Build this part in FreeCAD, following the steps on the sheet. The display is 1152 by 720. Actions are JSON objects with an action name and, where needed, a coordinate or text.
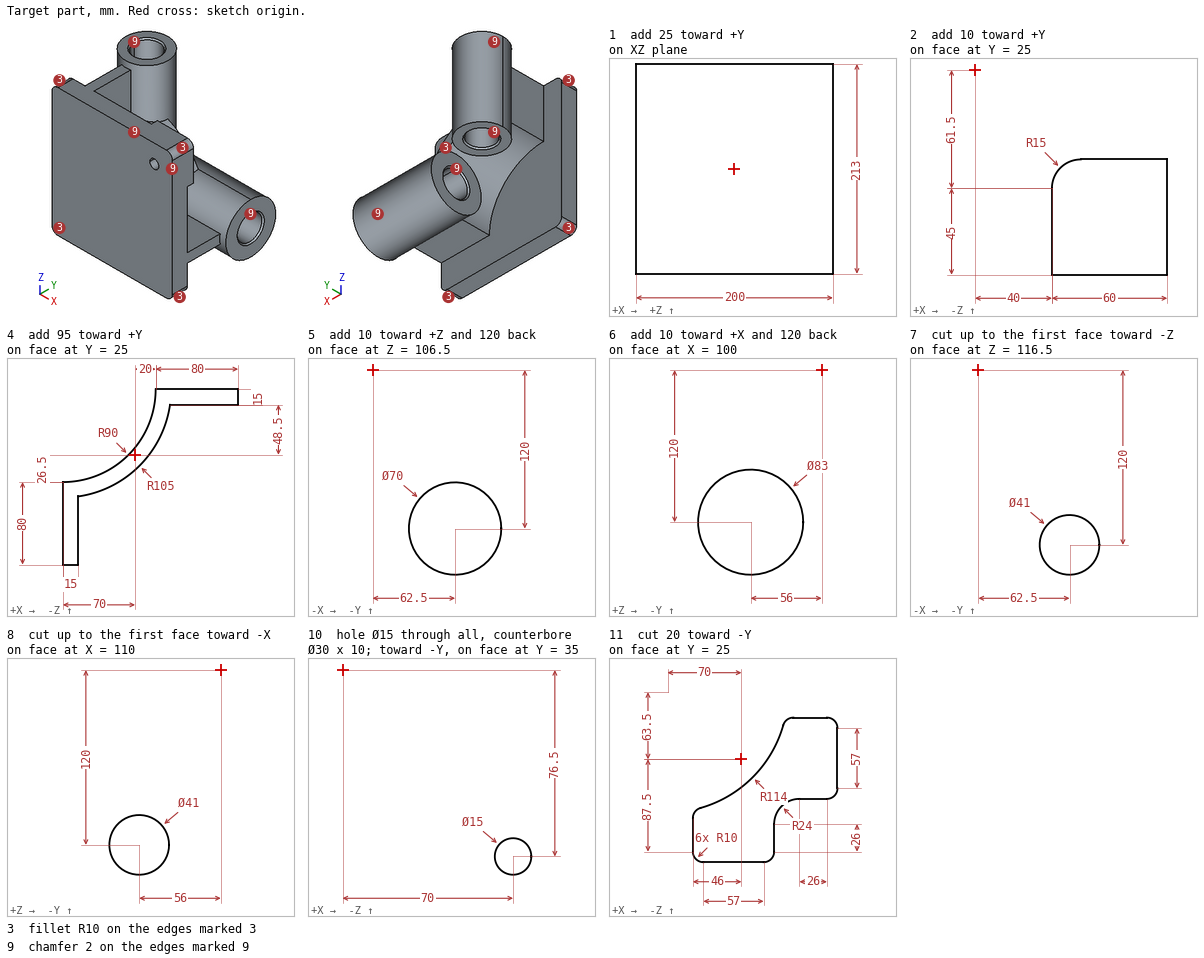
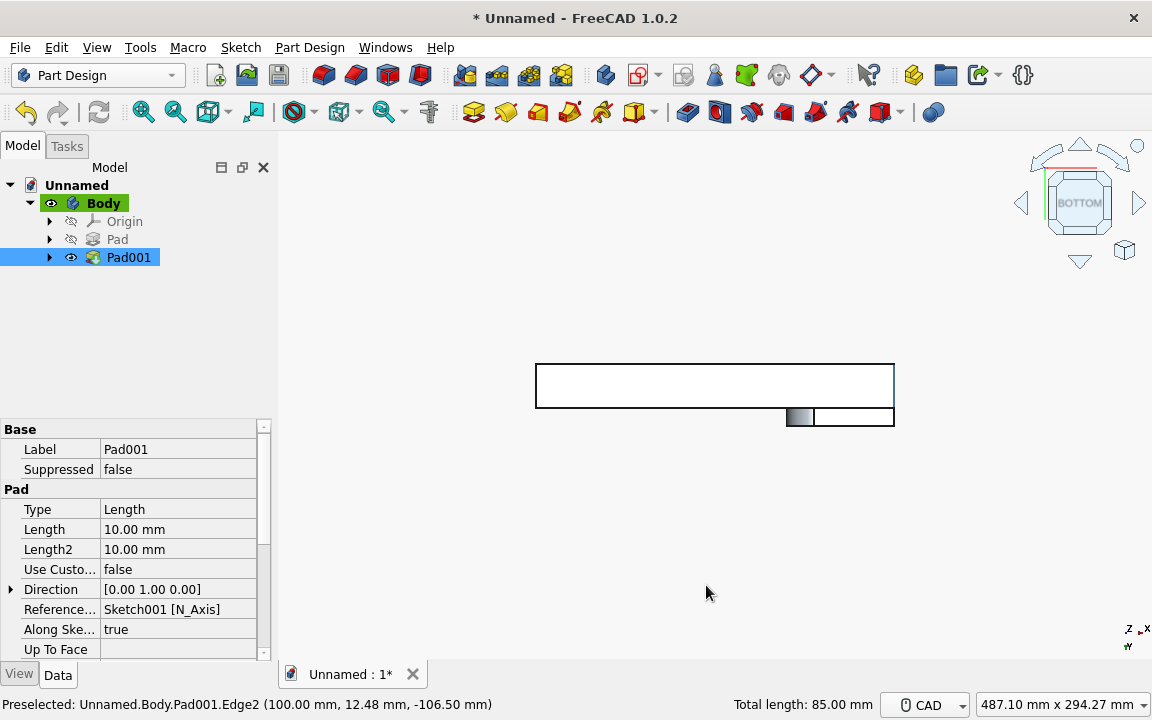
{"action": "left_click", "coordinate": [144, 112]}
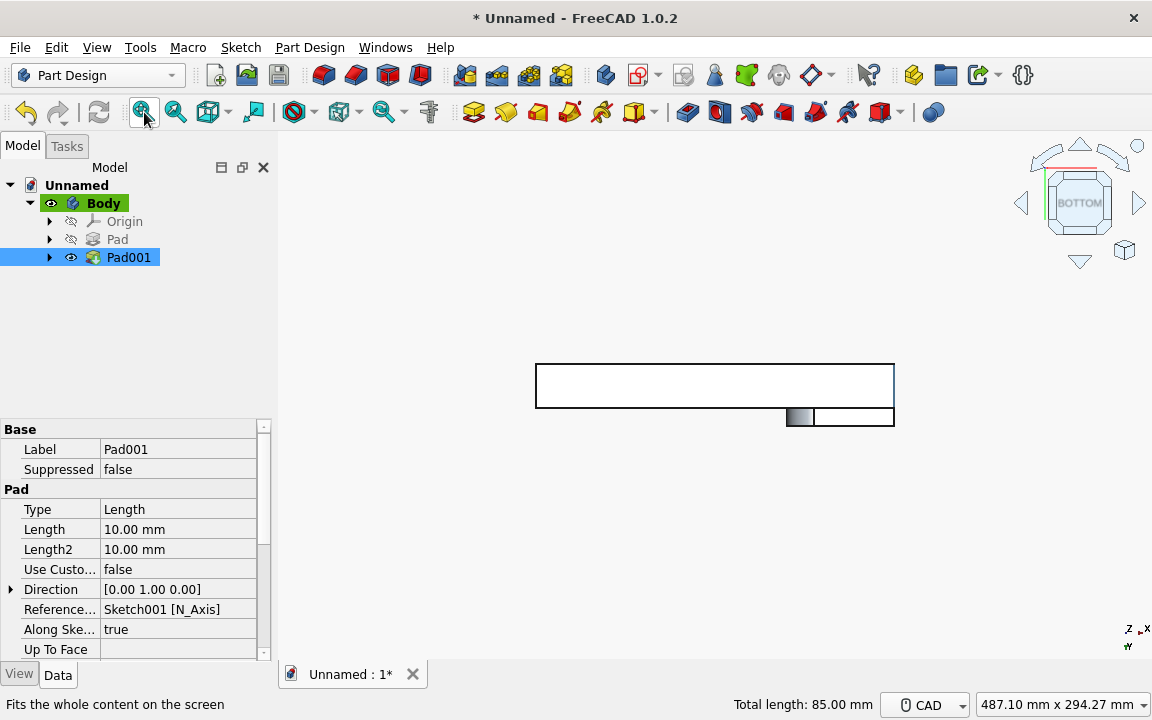
{"action": "left_click", "coordinate": [536, 385], "text": "ctrl"}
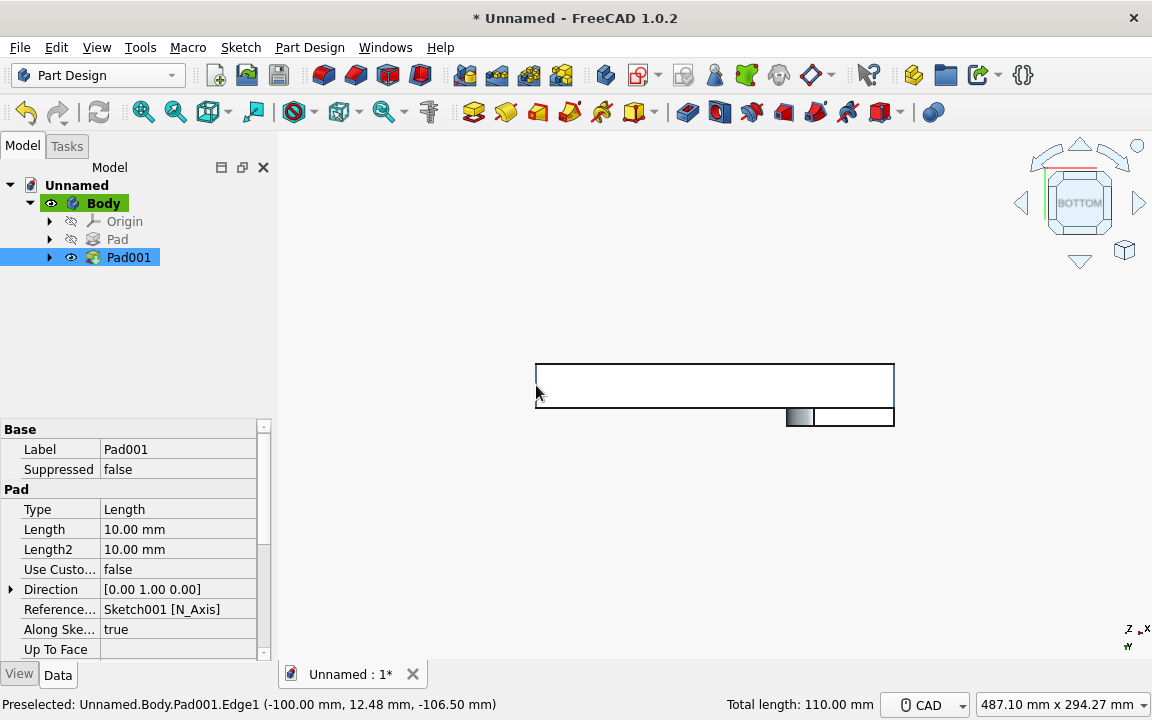
{"action": "left_click", "coordinate": [324, 76]}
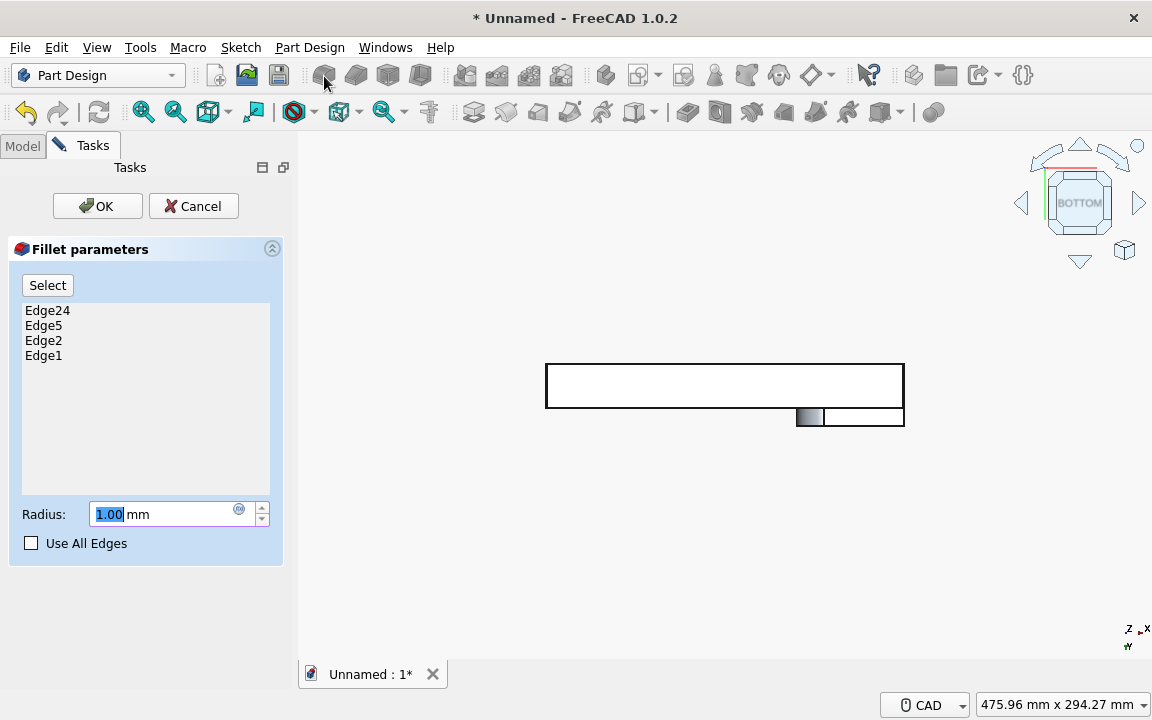
{"action": "type", "text": "10"}
{"action": "key", "text": "Tab"}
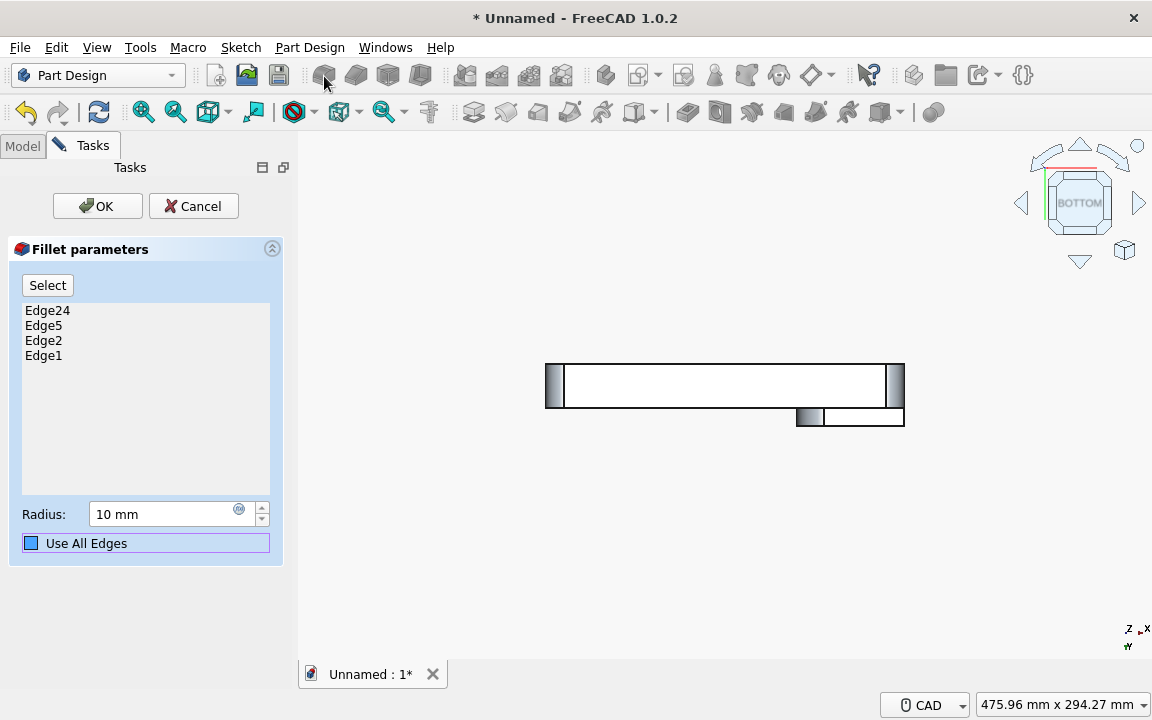
{"action": "left_click", "coordinate": [98, 206]}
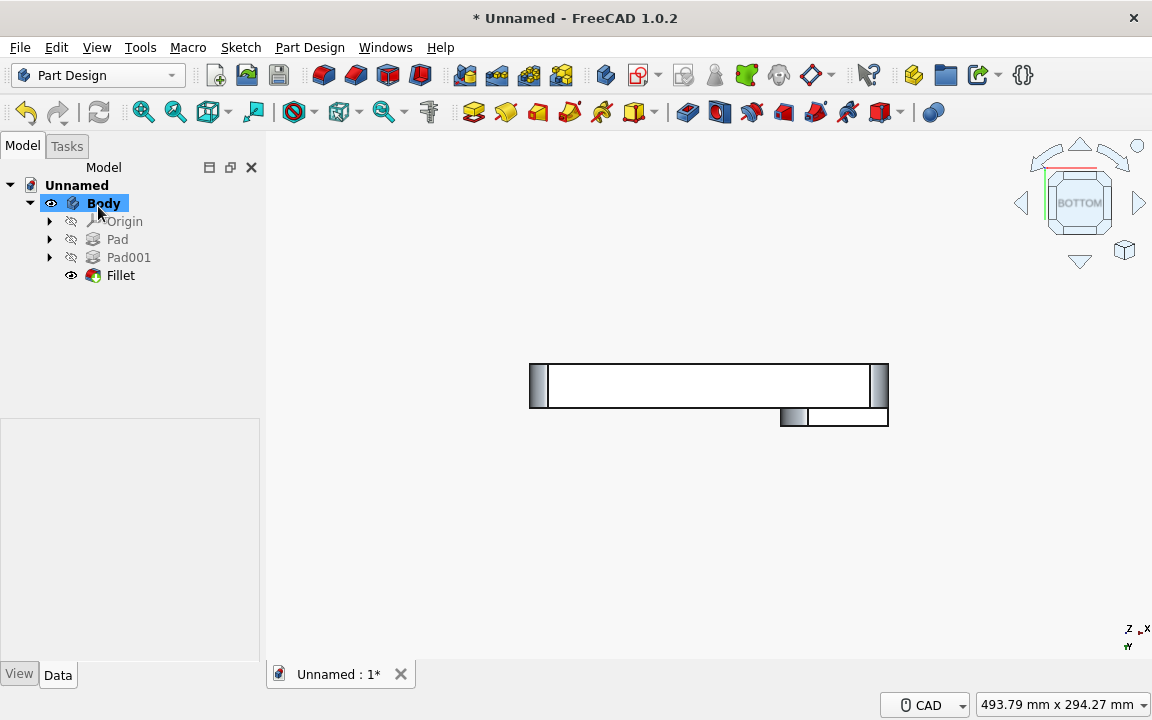
{"action": "left_click", "coordinate": [144, 112]}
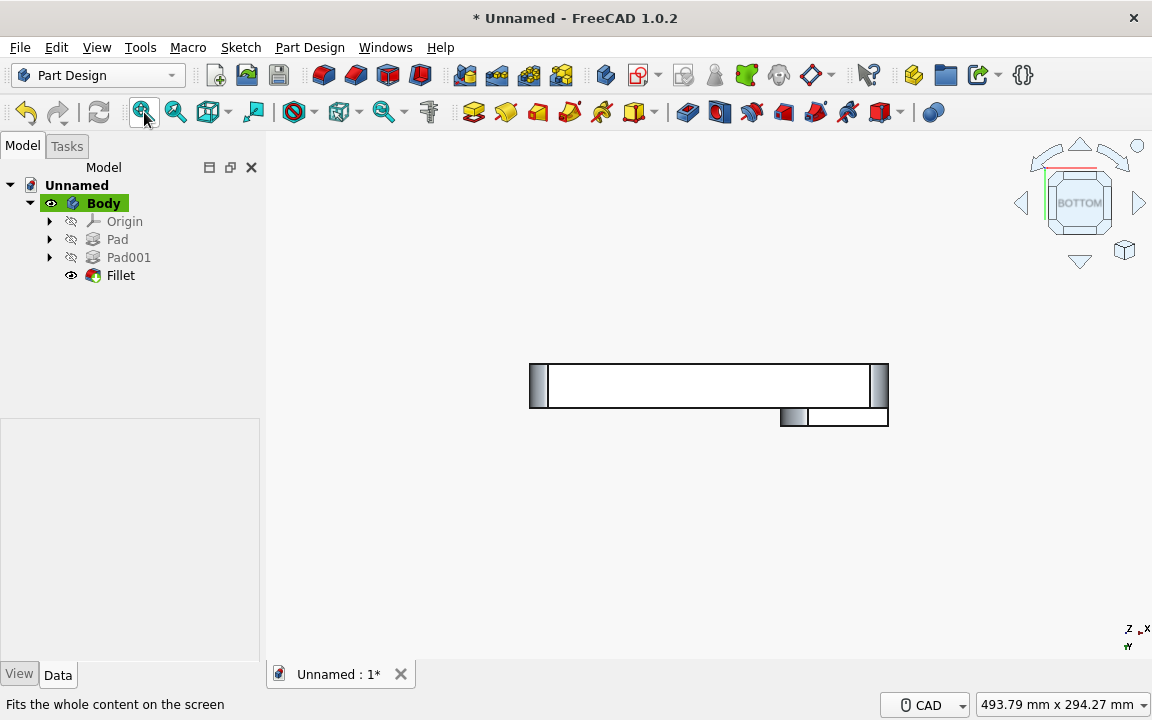
{"action": "key", "text": "4"}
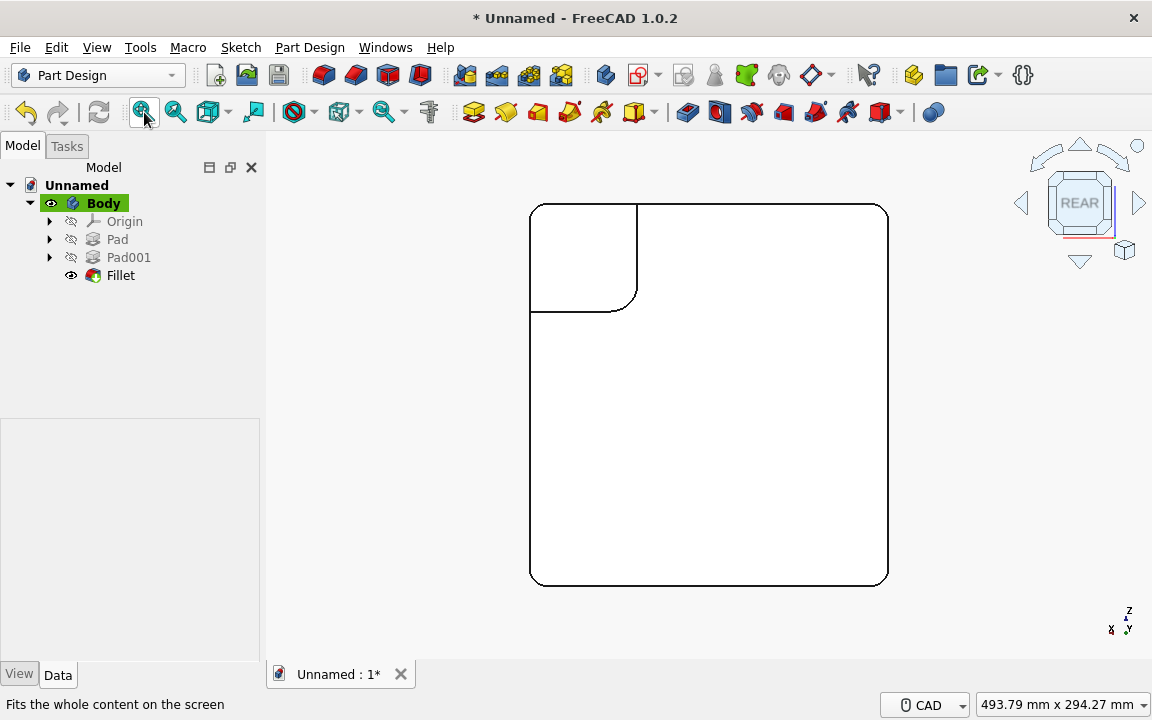
{"action": "left_click", "coordinate": [709, 449]}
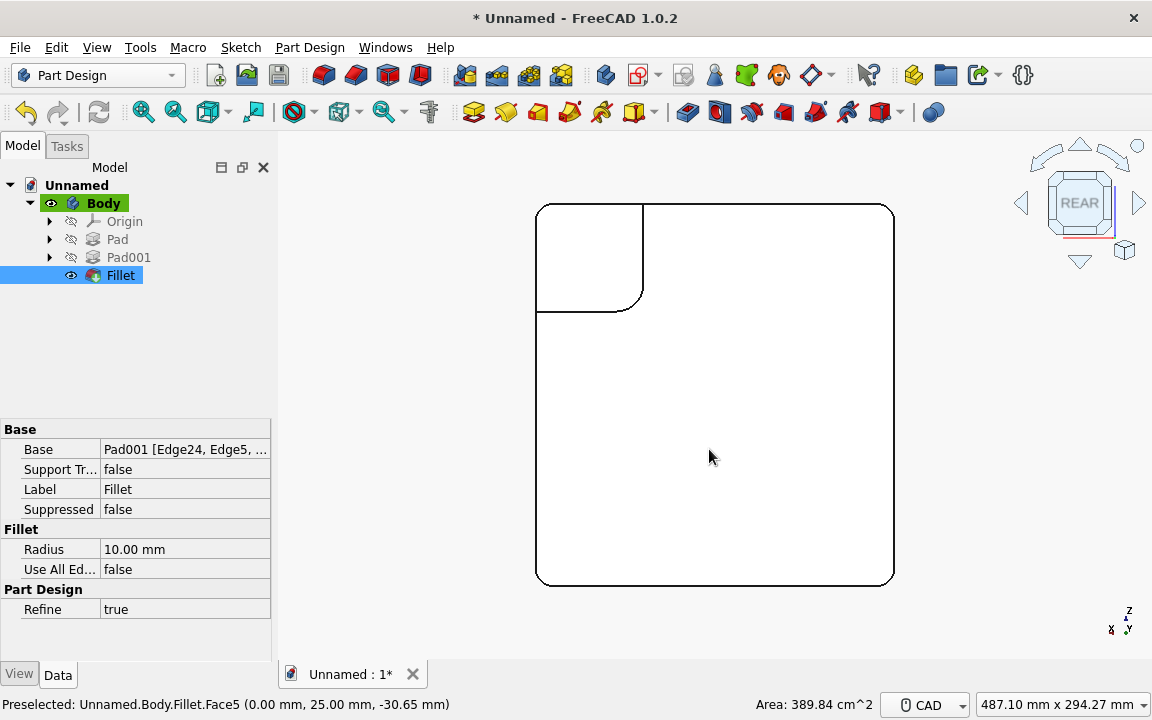
{"action": "left_click", "coordinate": [638, 76]}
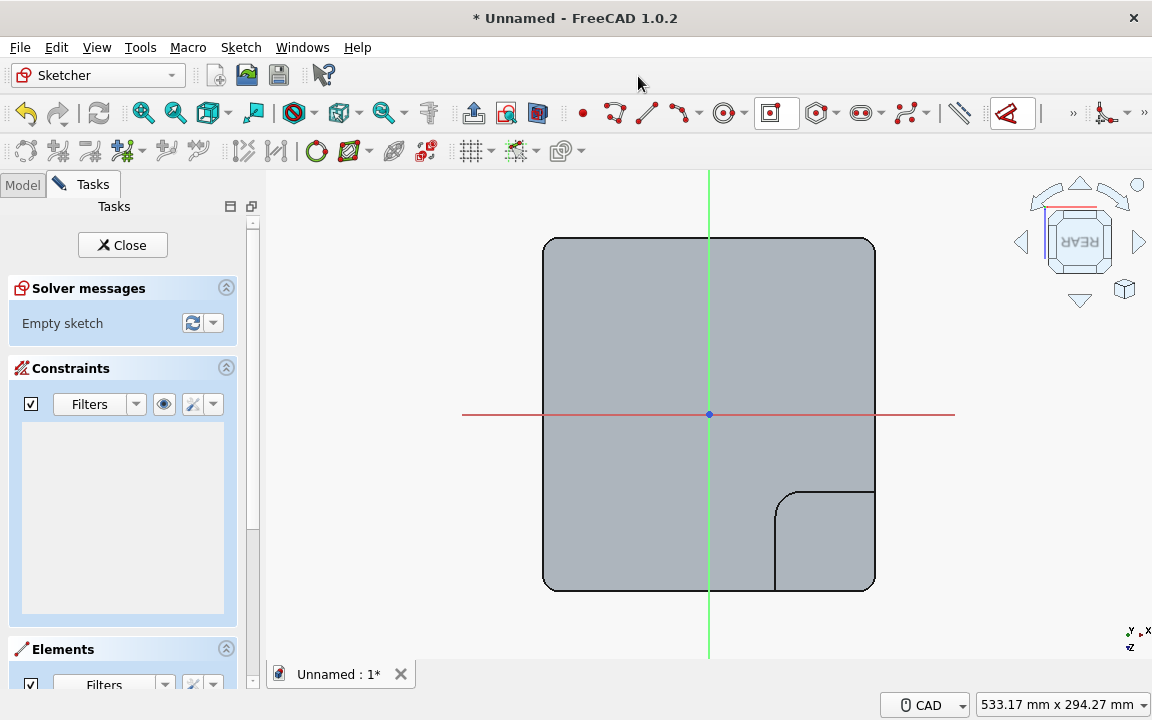
{"action": "left_click", "coordinate": [538, 114]}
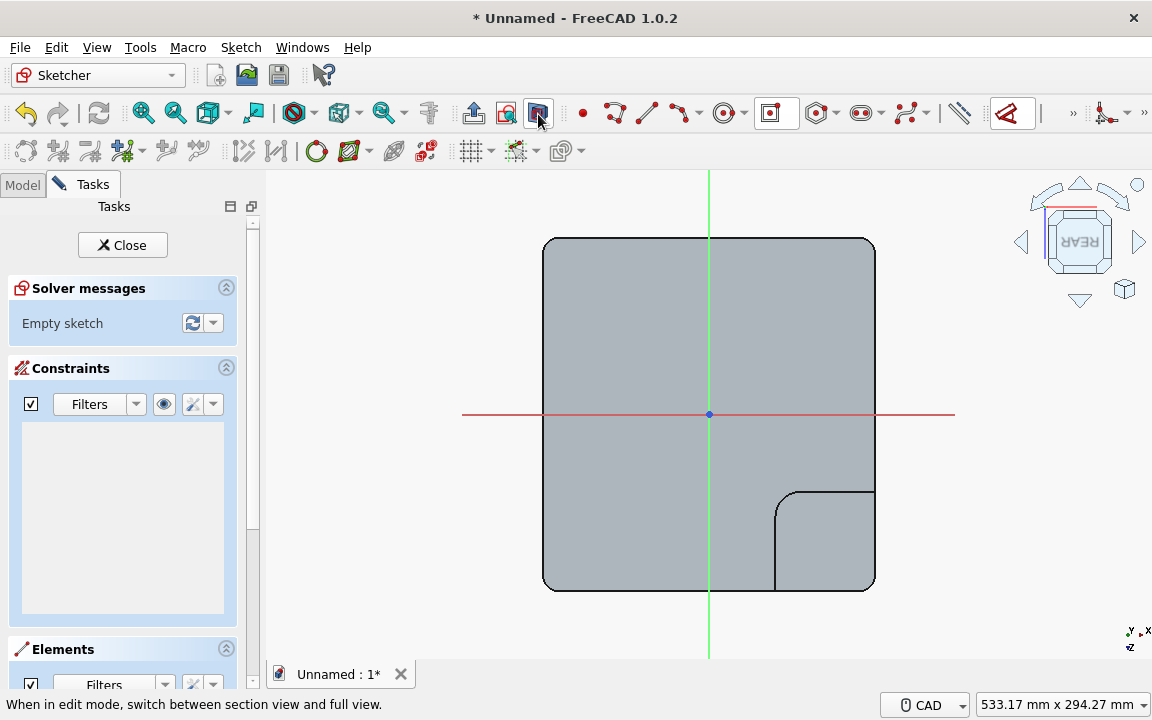
{"action": "left_click", "coordinate": [616, 114]}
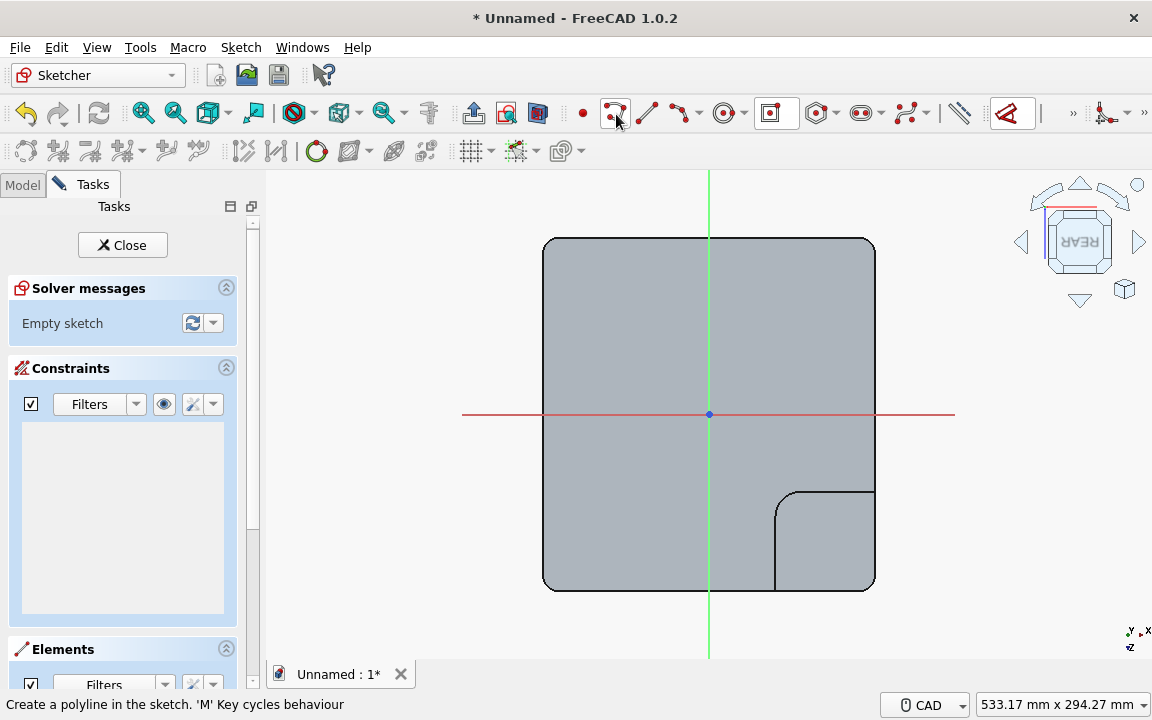
{"action": "left_click", "coordinate": [593, 459]}
{"action": "left_click", "coordinate": [593, 591]}
{"action": "left_click", "coordinate": [618, 591]}
{"action": "left_click", "coordinate": [618, 482]}
{"action": "right_click", "coordinate": [618, 482]}